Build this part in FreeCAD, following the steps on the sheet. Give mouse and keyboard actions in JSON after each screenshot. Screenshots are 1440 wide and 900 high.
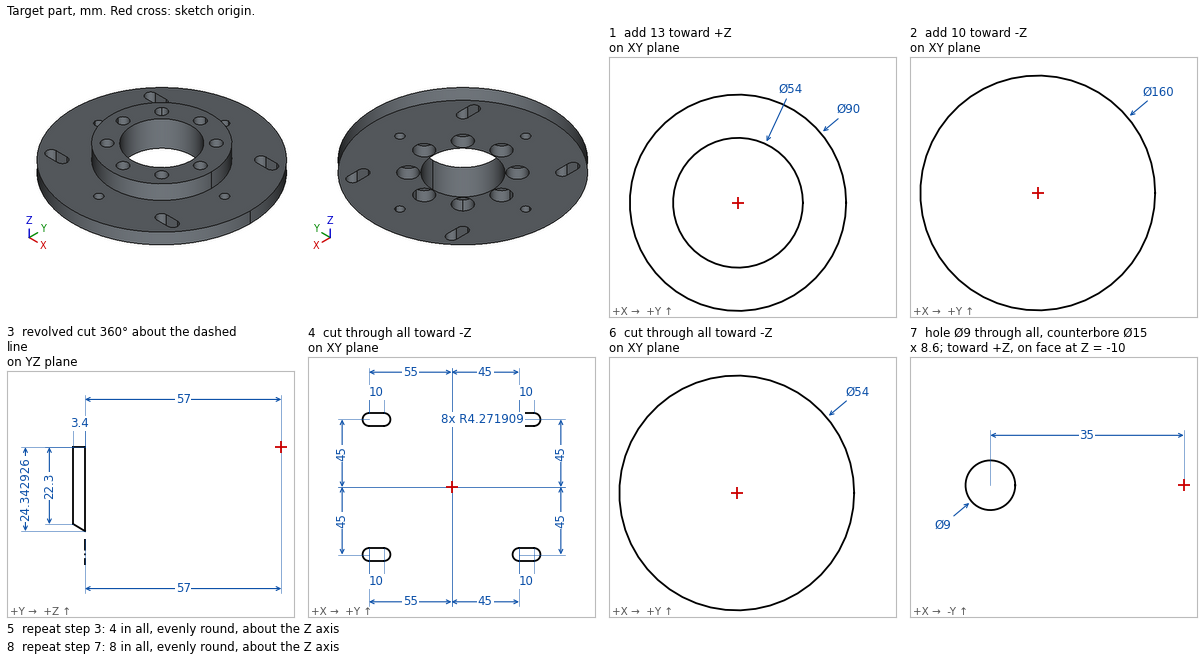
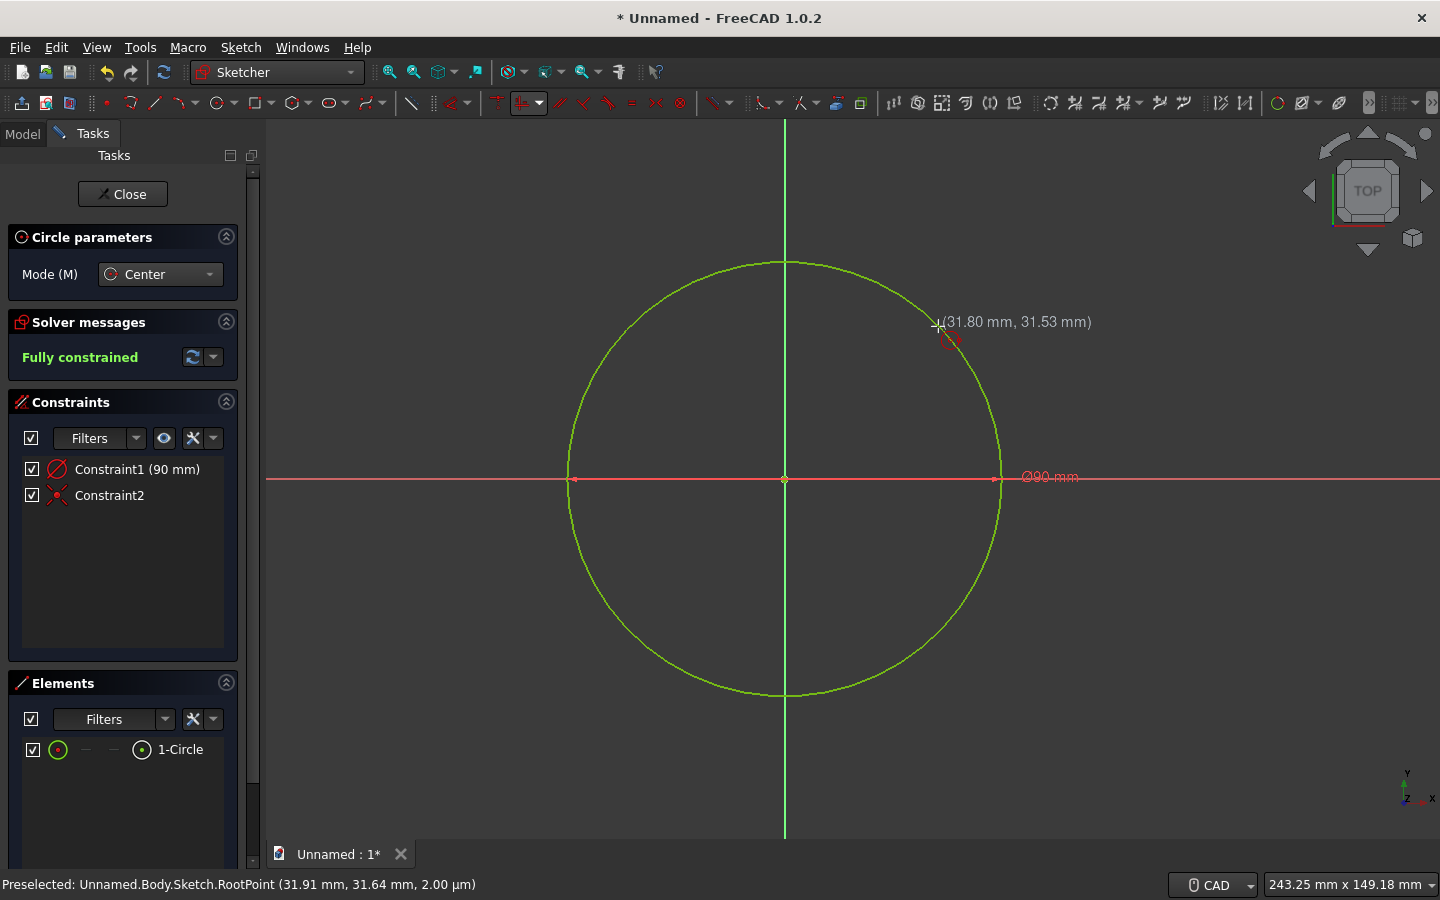
{"action": "left_click", "coordinate": [785, 479]}
{"action": "mouse_move", "coordinate": [877, 387]}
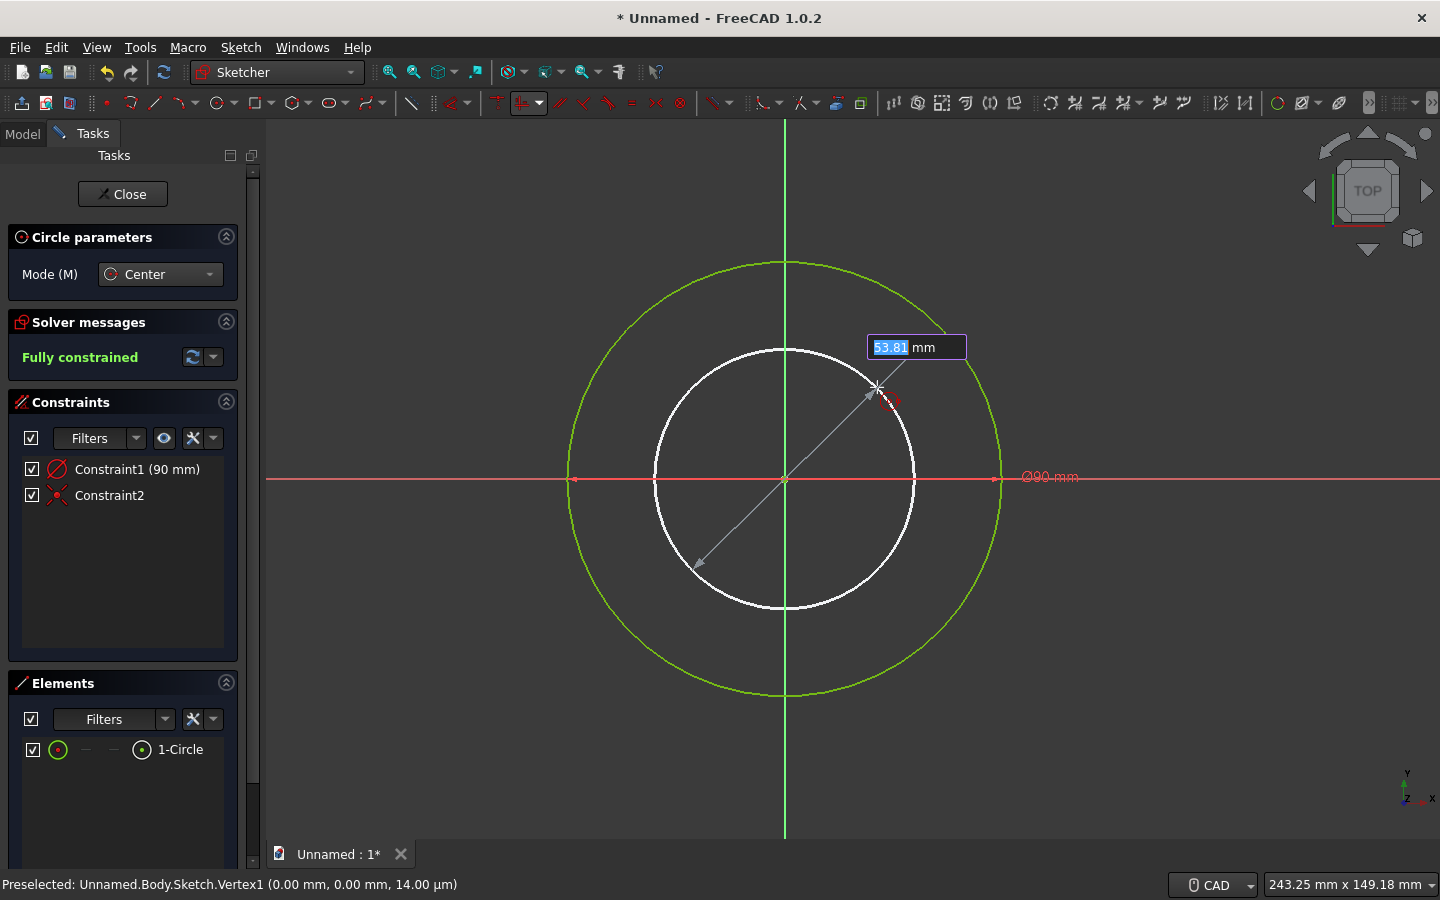
{"action": "type", "text": "54"}
{"action": "key", "text": "Return"}
{"action": "key", "text": "Escape"}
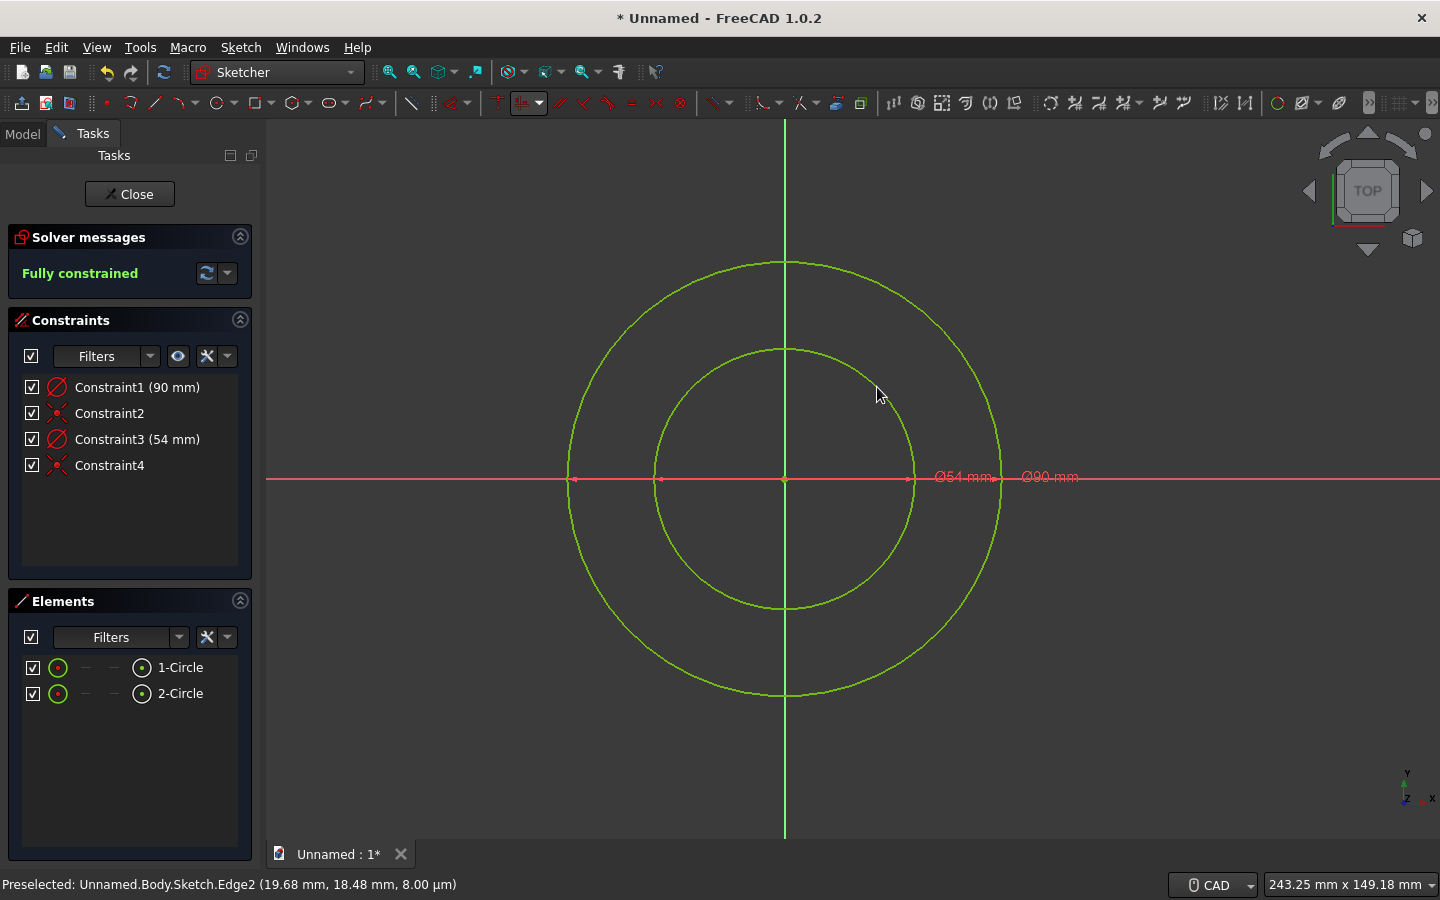
{"action": "left_click", "coordinate": [130, 194]}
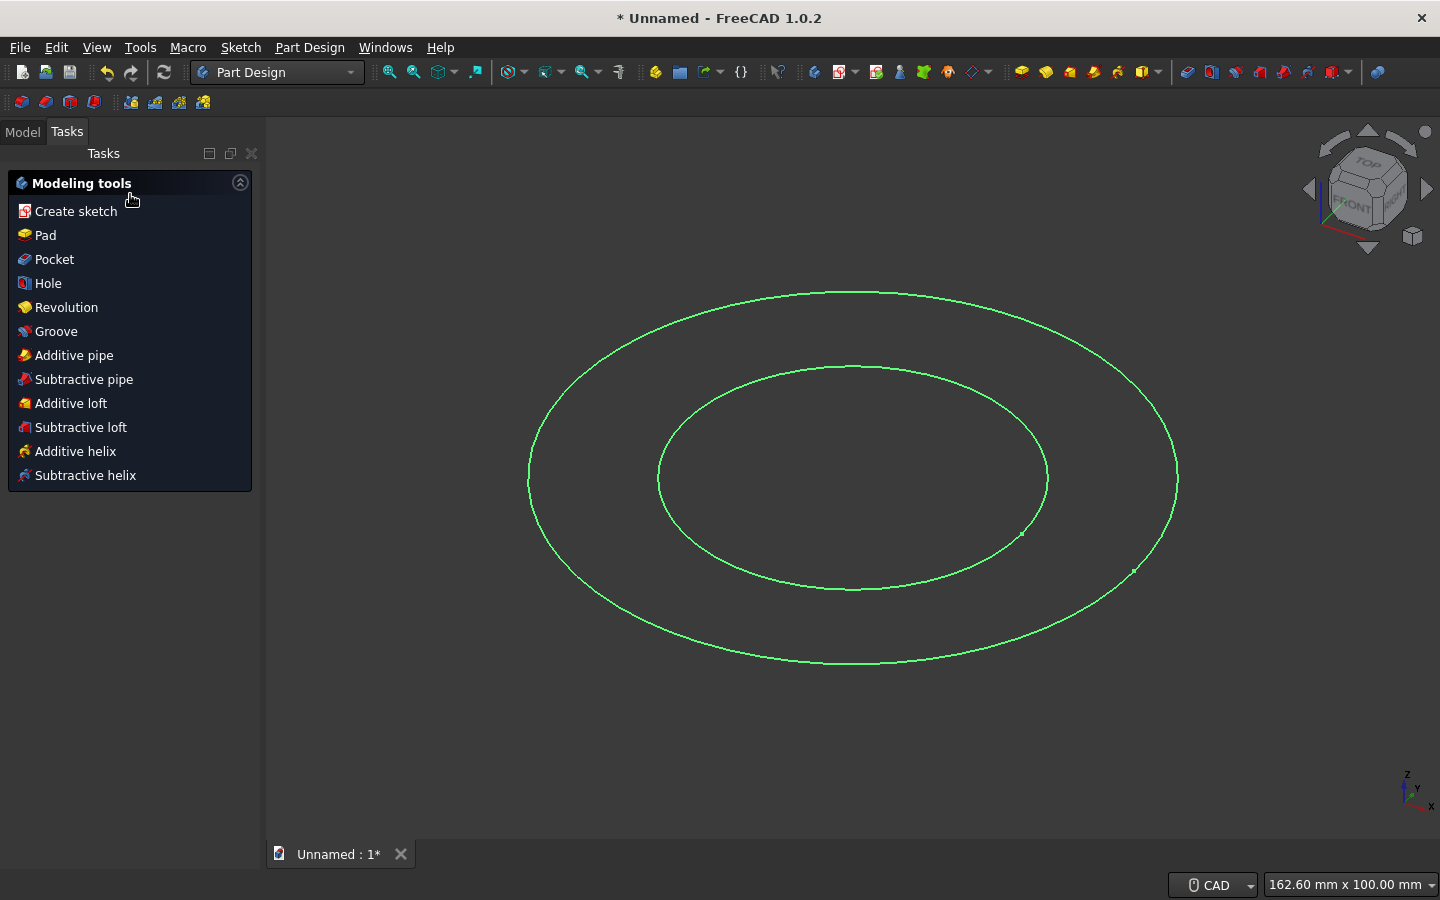
{"action": "left_click", "coordinate": [1022, 72]}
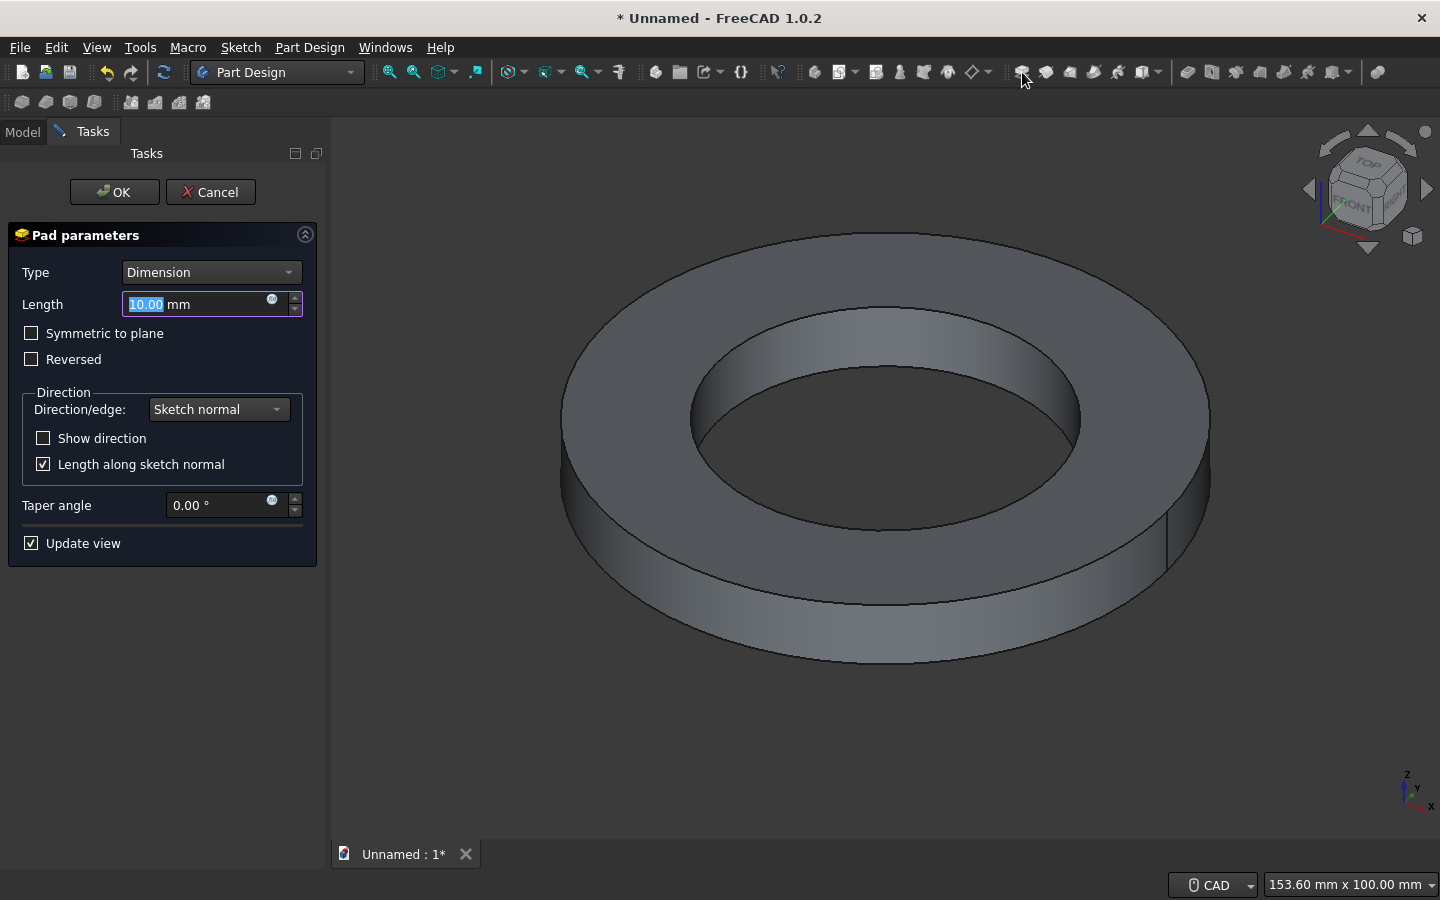
{"action": "type", "text": "13"}
{"action": "key", "text": "Tab"}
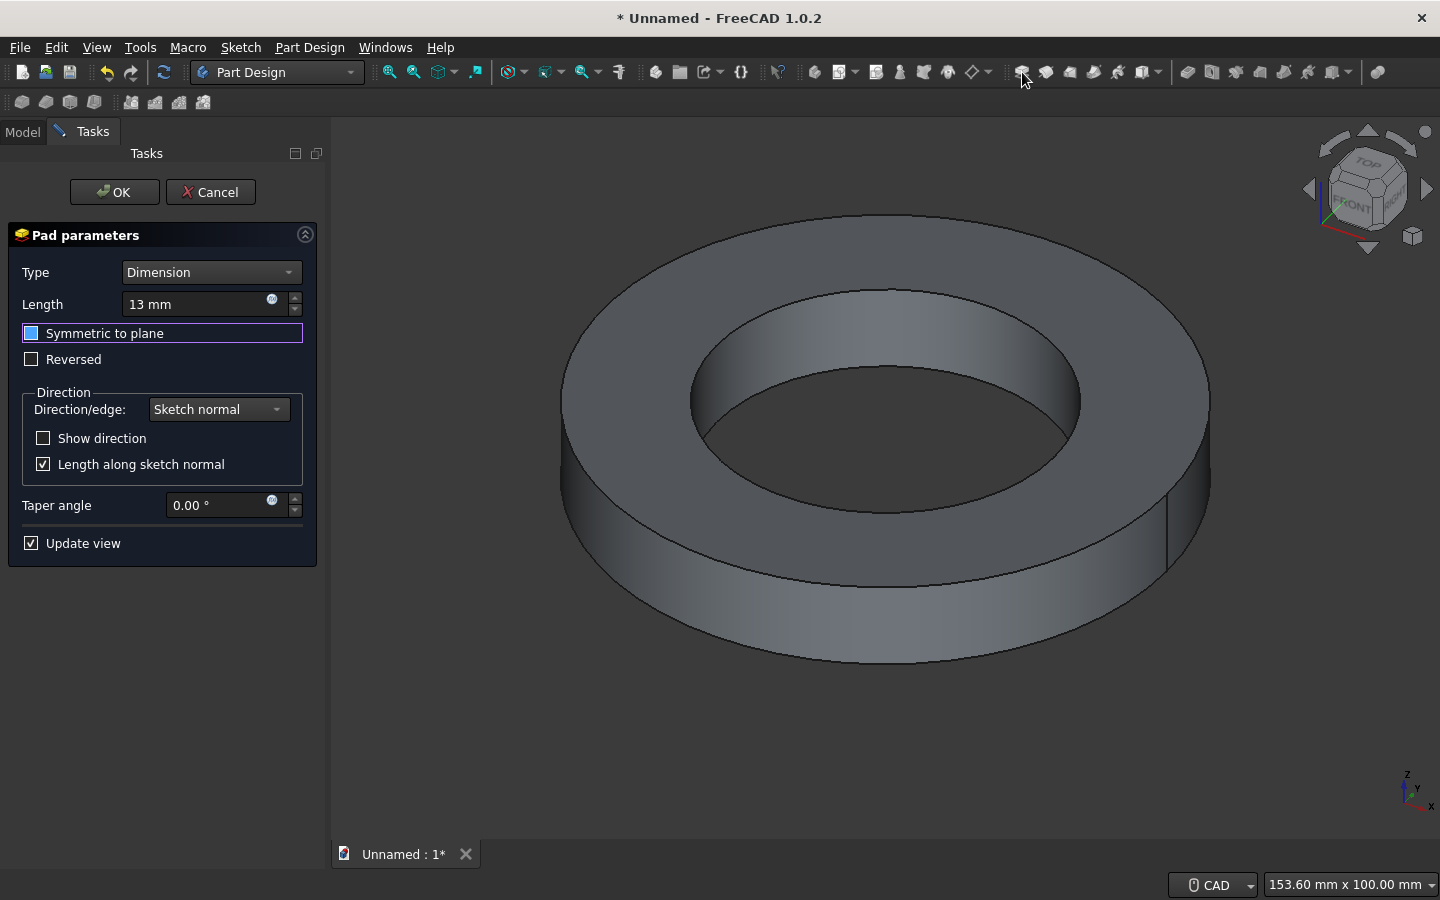
{"action": "left_click", "coordinate": [115, 192]}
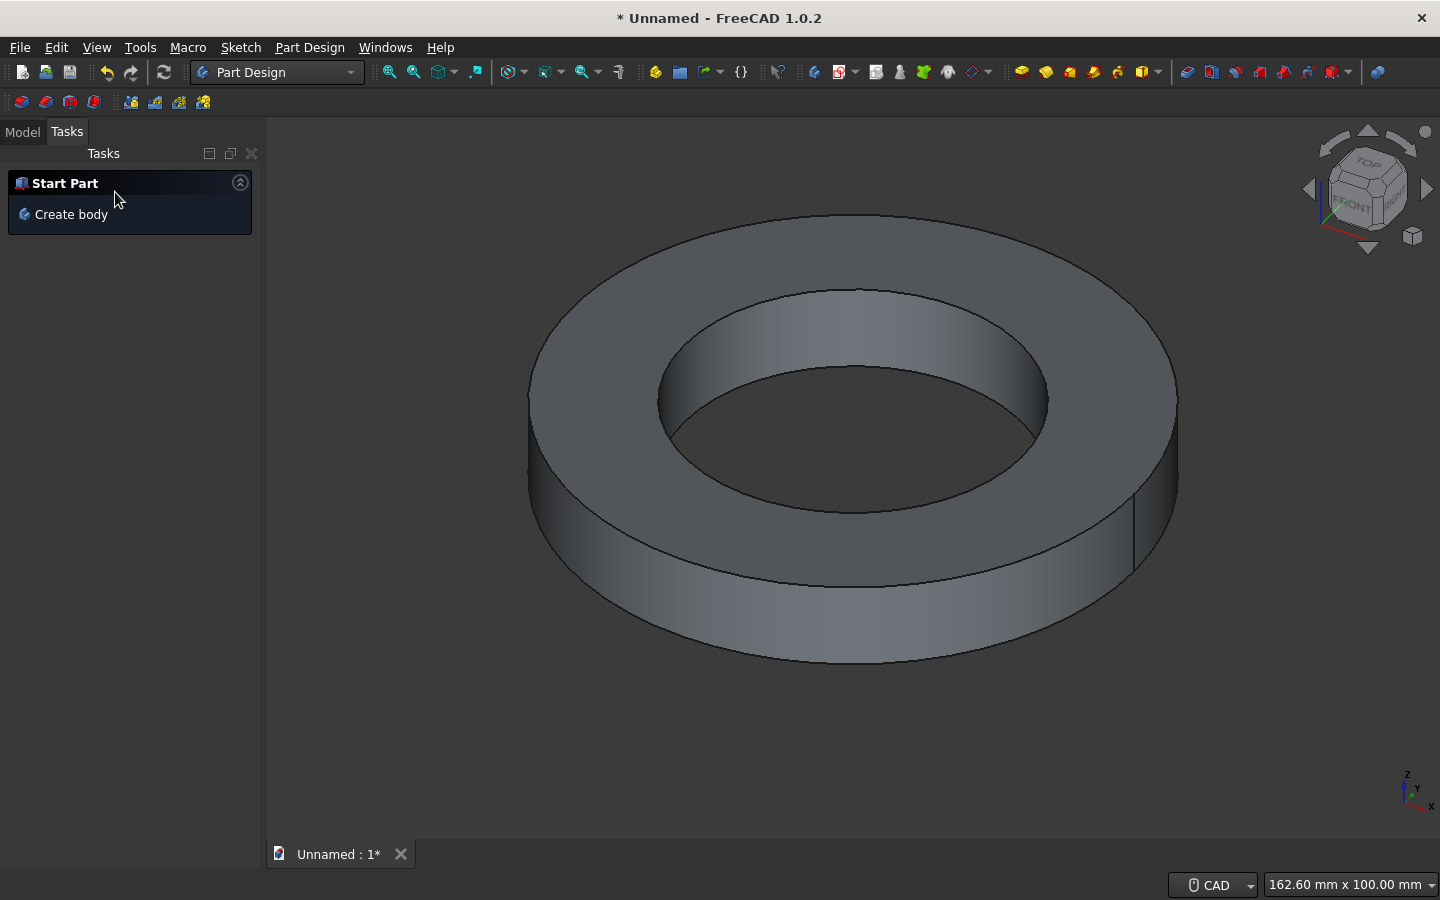
{"action": "left_click", "coordinate": [840, 72]}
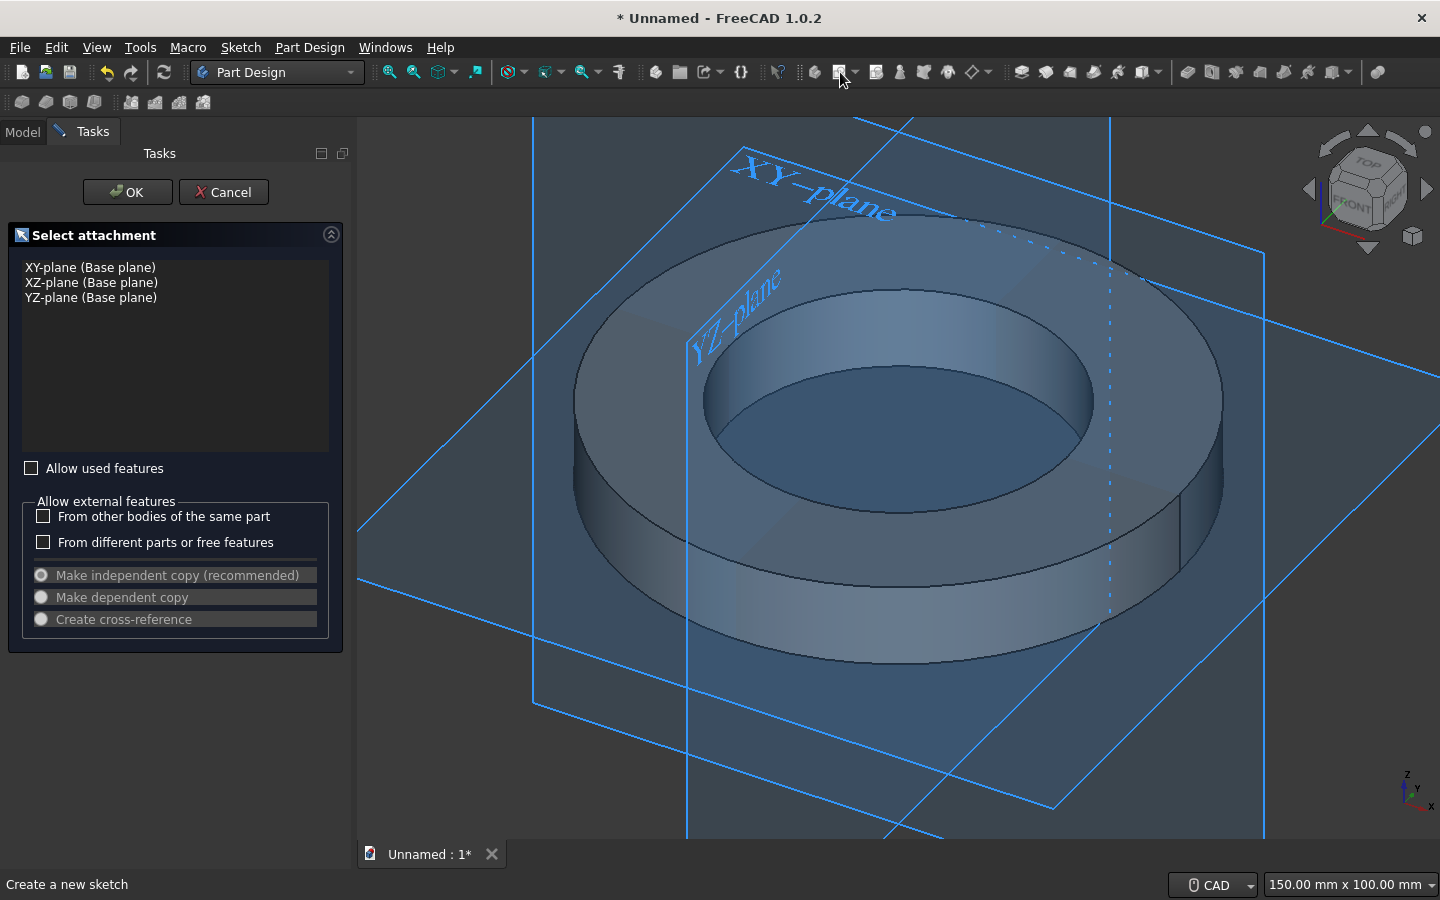
{"action": "left_click", "coordinate": [82, 268]}